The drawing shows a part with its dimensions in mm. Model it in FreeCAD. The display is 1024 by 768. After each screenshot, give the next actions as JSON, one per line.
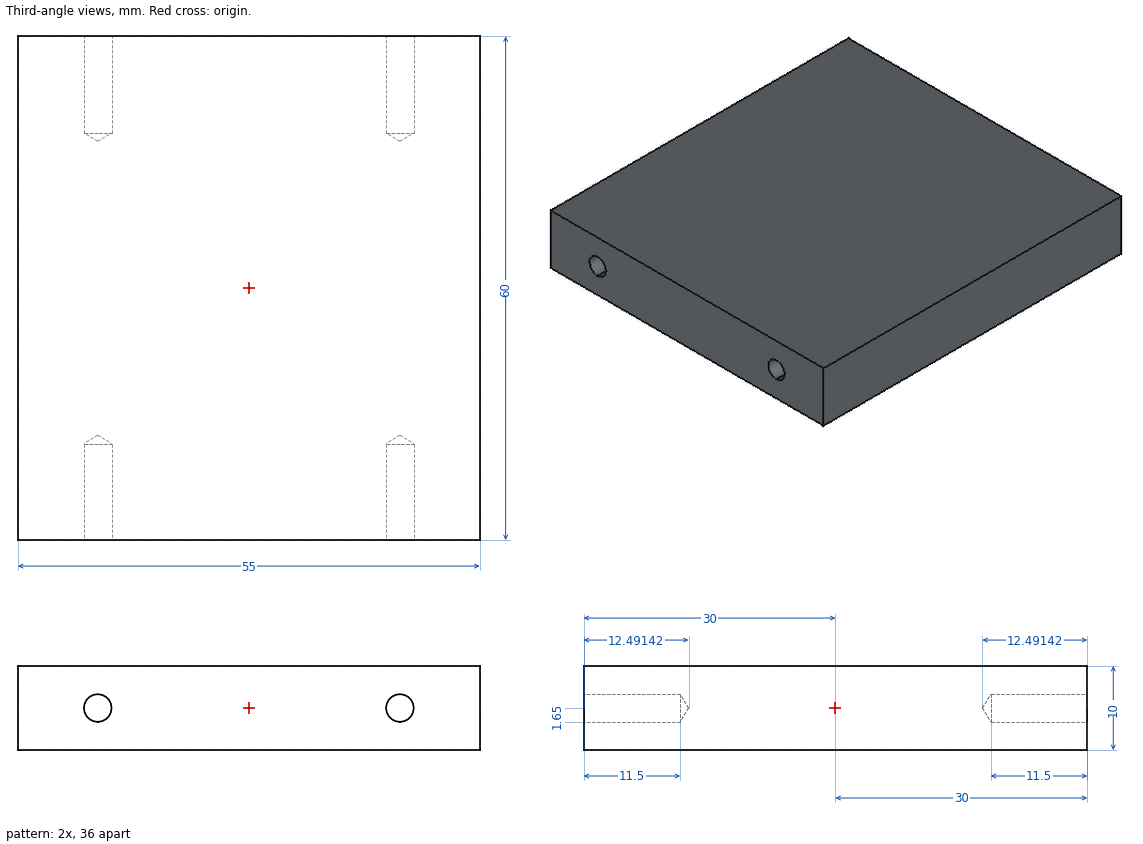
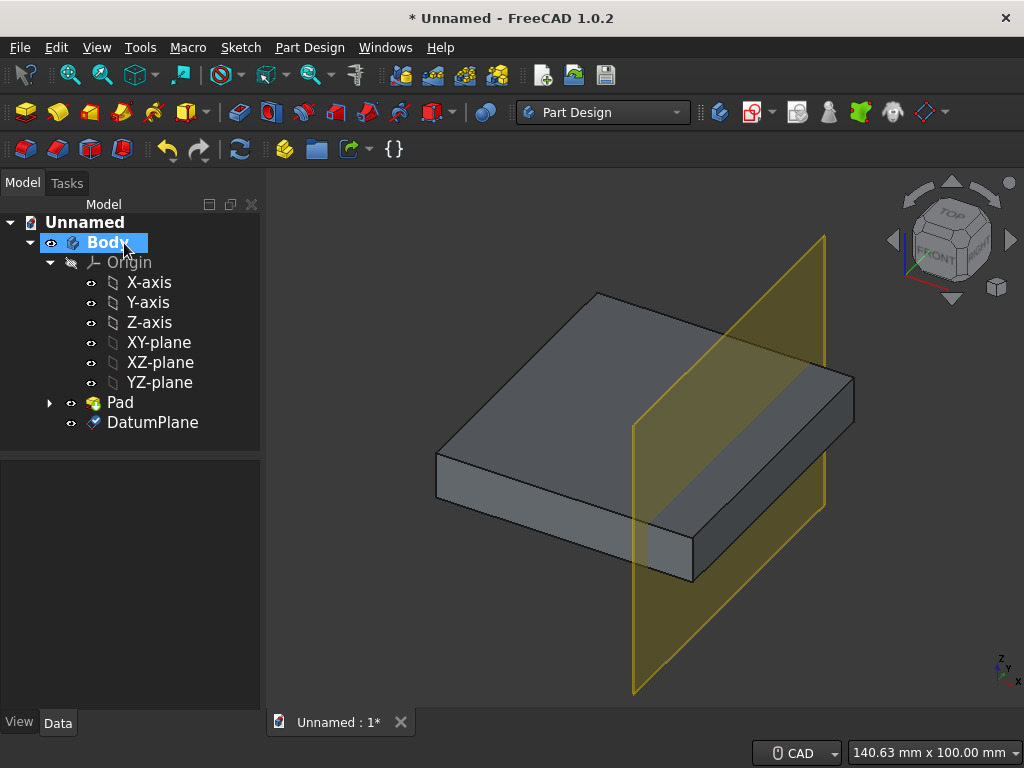
{"action": "left_click", "coordinate": [116, 423]}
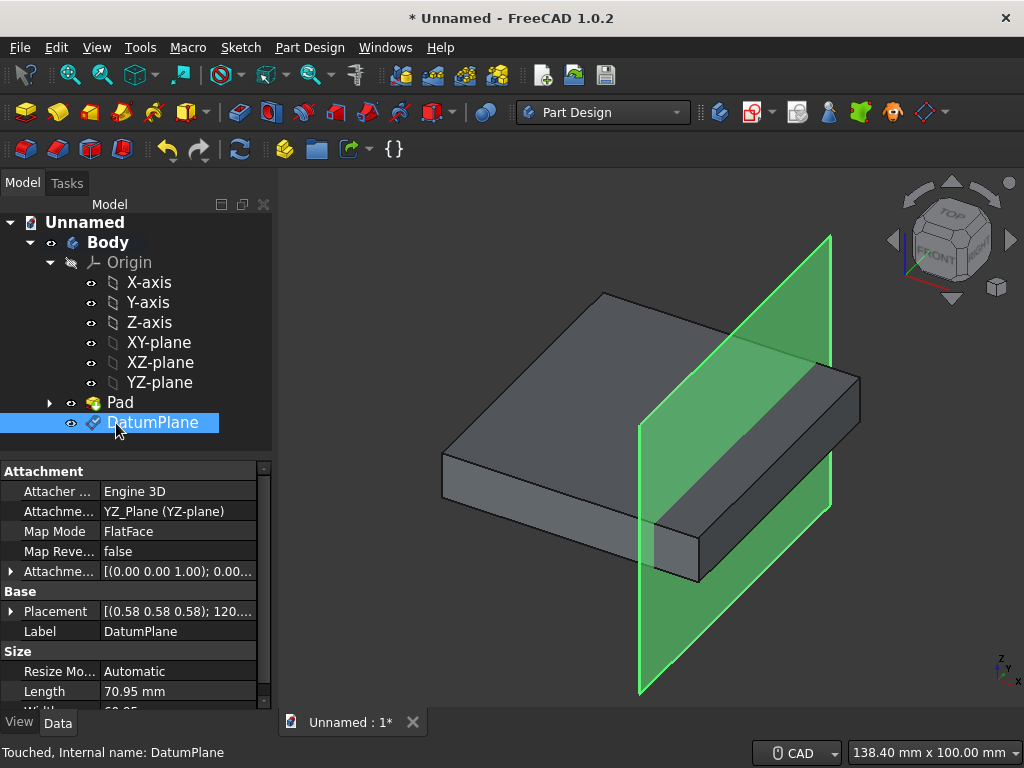
{"action": "left_click", "coordinate": [752, 112]}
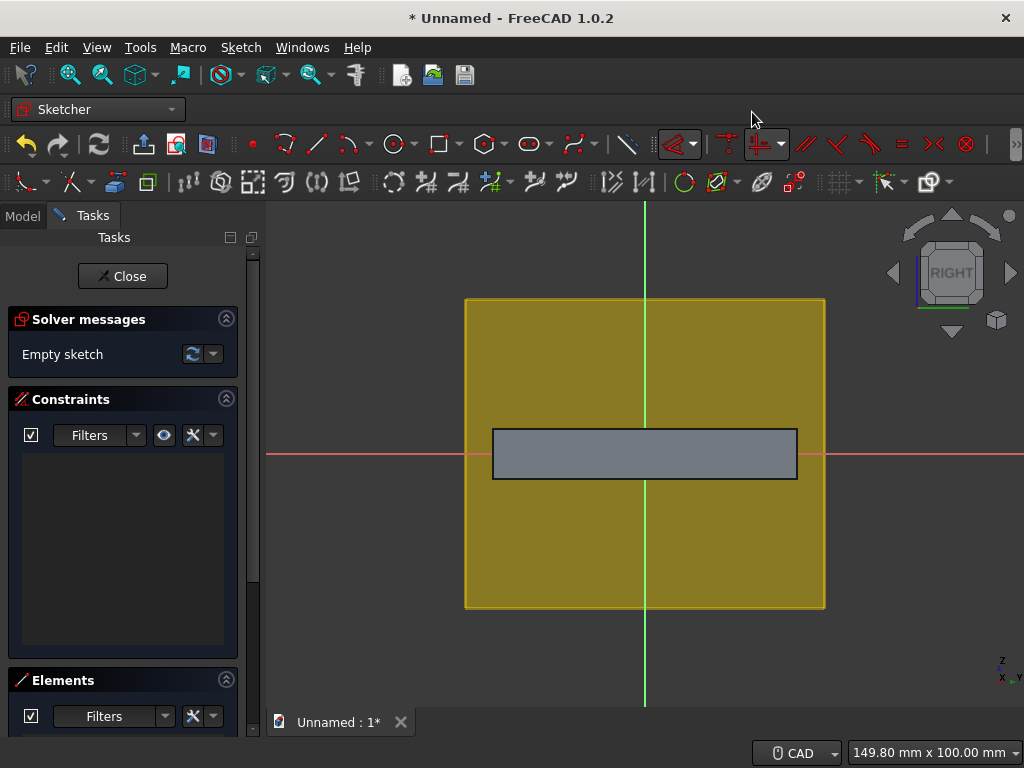
{"action": "left_click", "coordinate": [208, 144]}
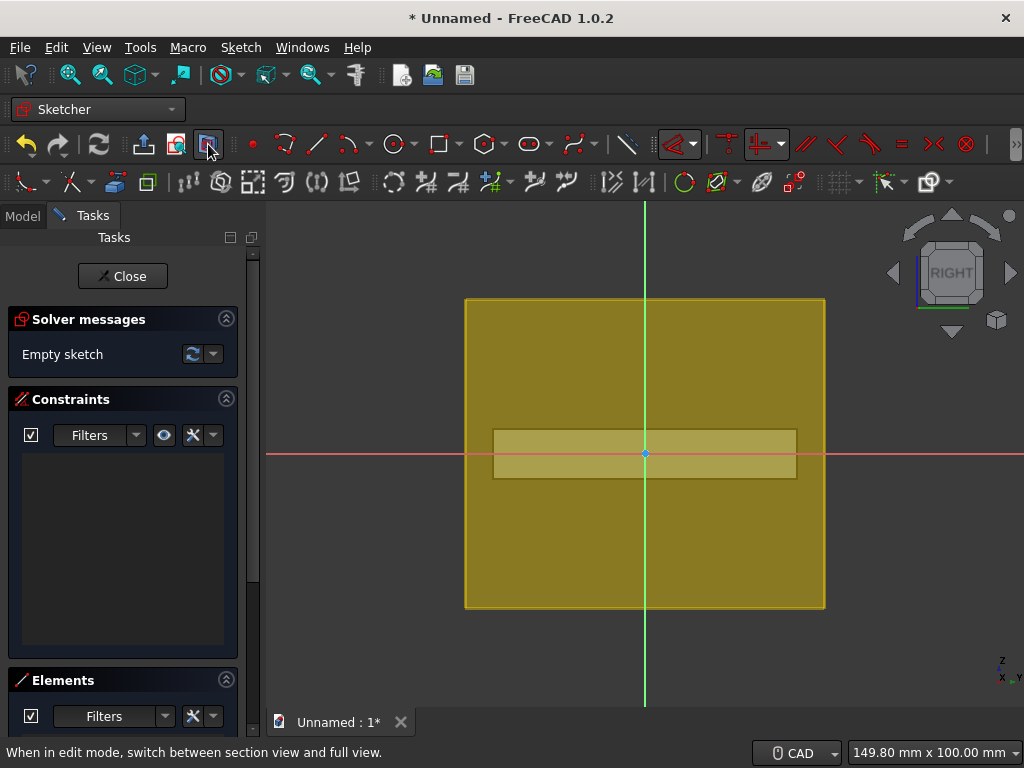
{"action": "scroll", "coordinate": [565, 461], "scroll_direction": "up", "scroll_amount": 5}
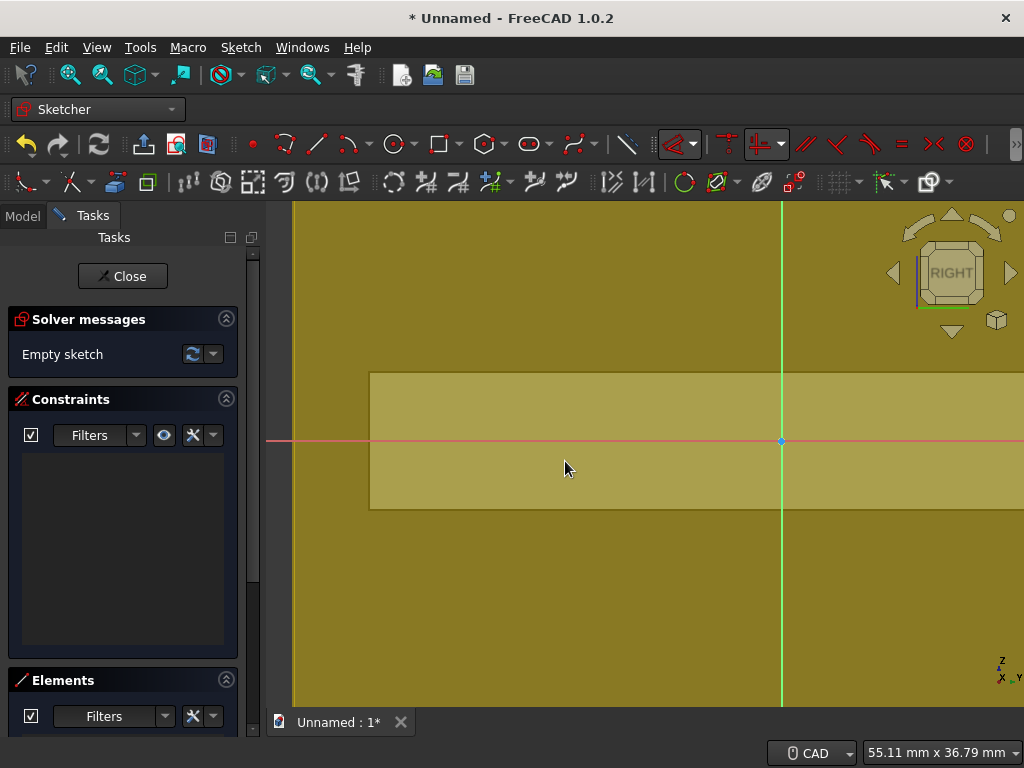
{"action": "key", "text": "g m"}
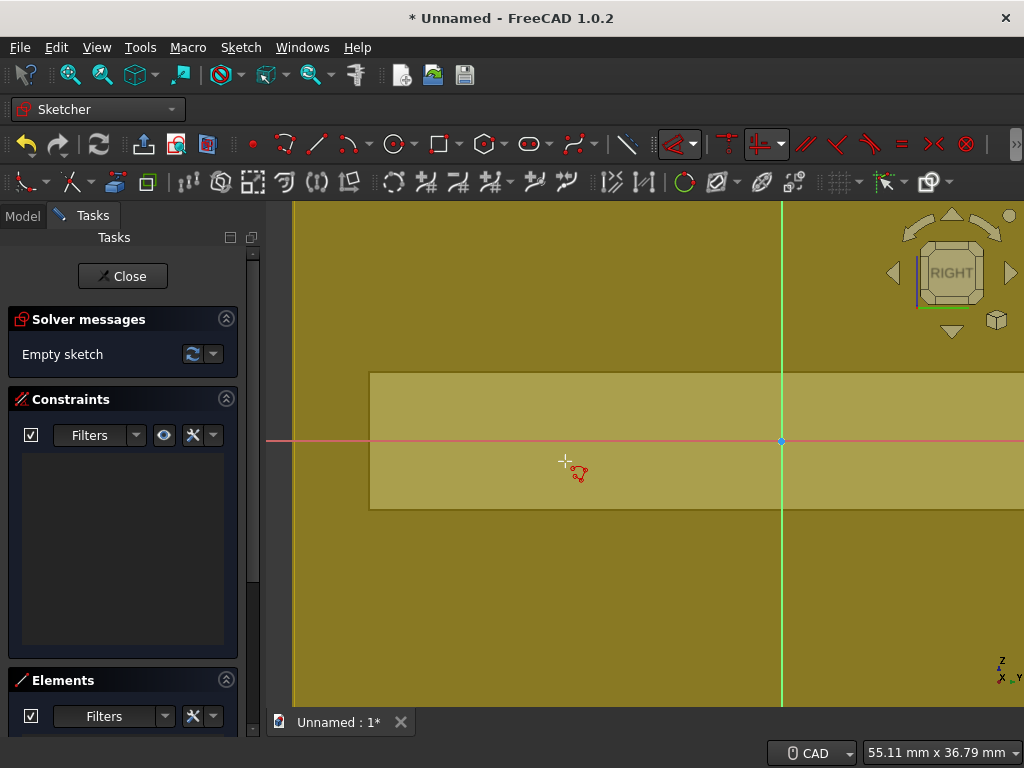
{"action": "left_click", "coordinate": [541, 441]}
{"action": "left_click", "coordinate": [369, 450]}
{"action": "left_click", "coordinate": [369, 464]}
{"action": "left_click", "coordinate": [527, 464]}
{"action": "left_click", "coordinate": [541, 441]}
{"action": "key", "text": "Escape"}
{"action": "key", "text": "Escape"}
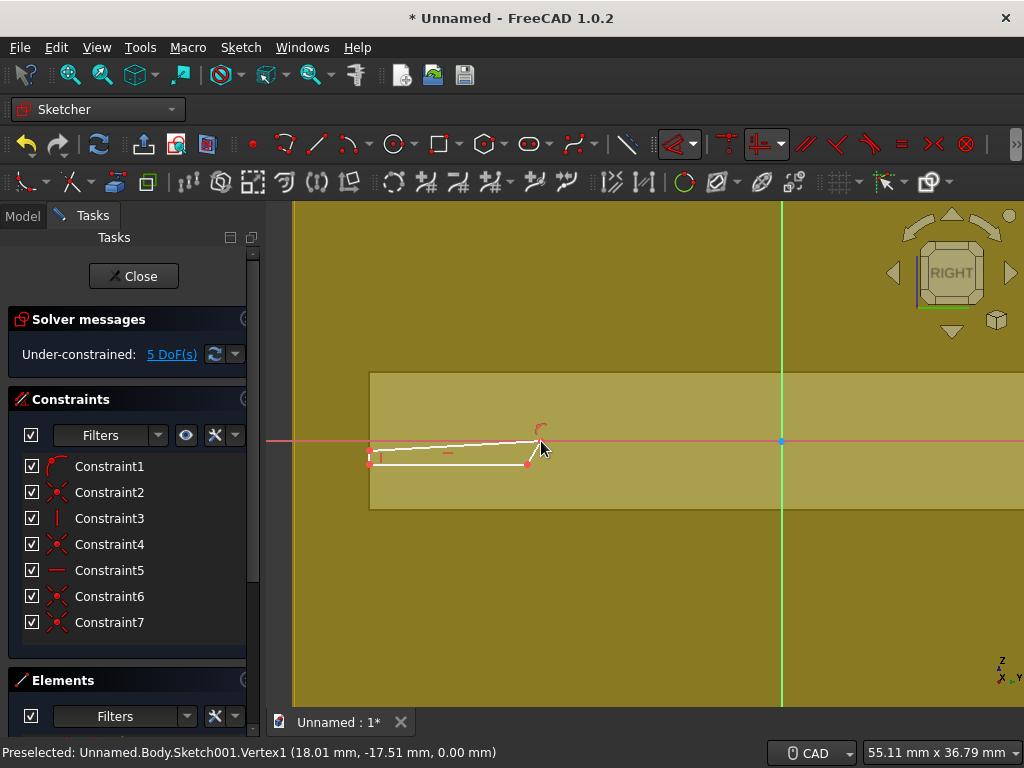
{"action": "left_click", "coordinate": [489, 444]}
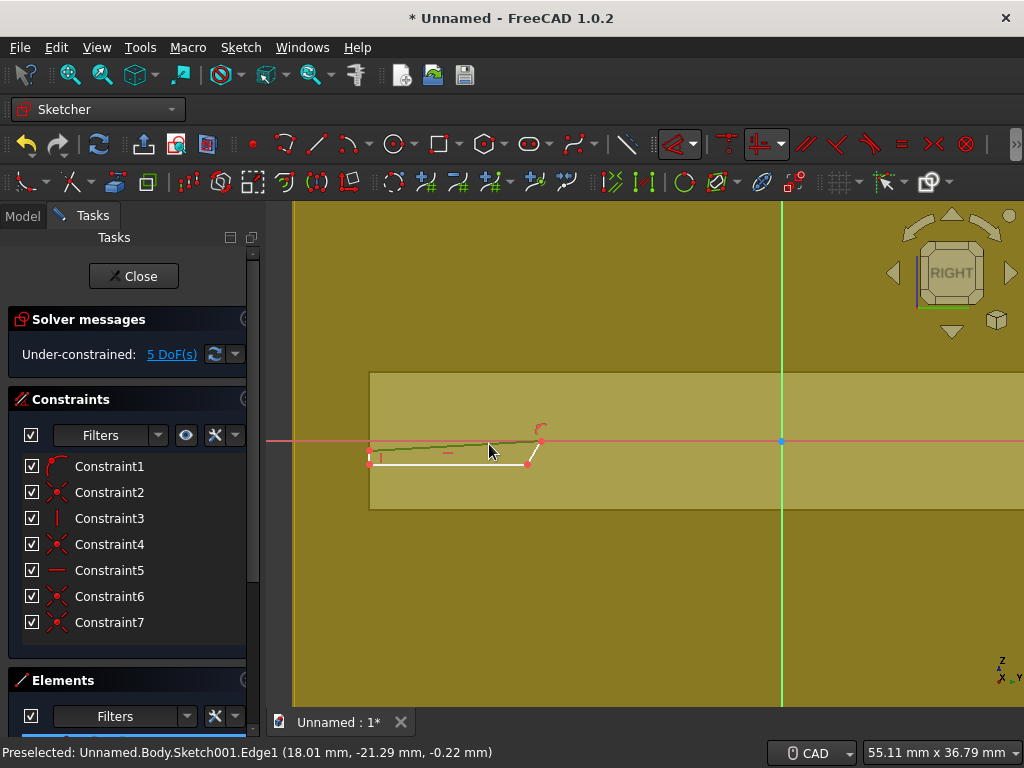
{"action": "key", "text": "h"}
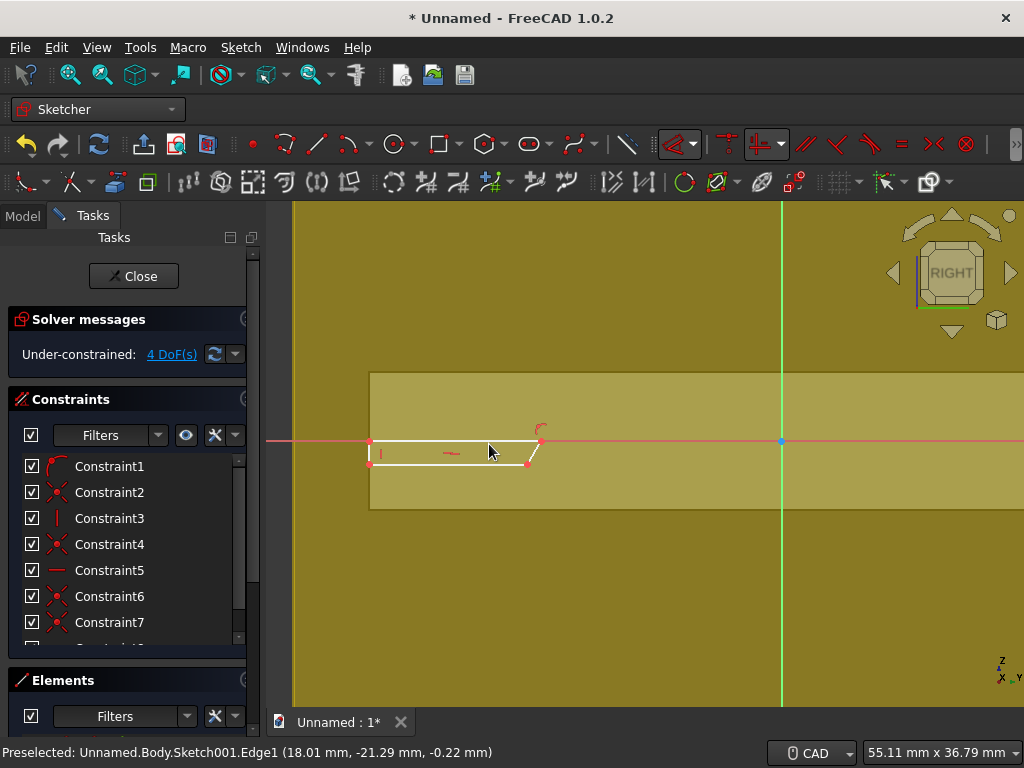
{"action": "left_click", "coordinate": [674, 144]}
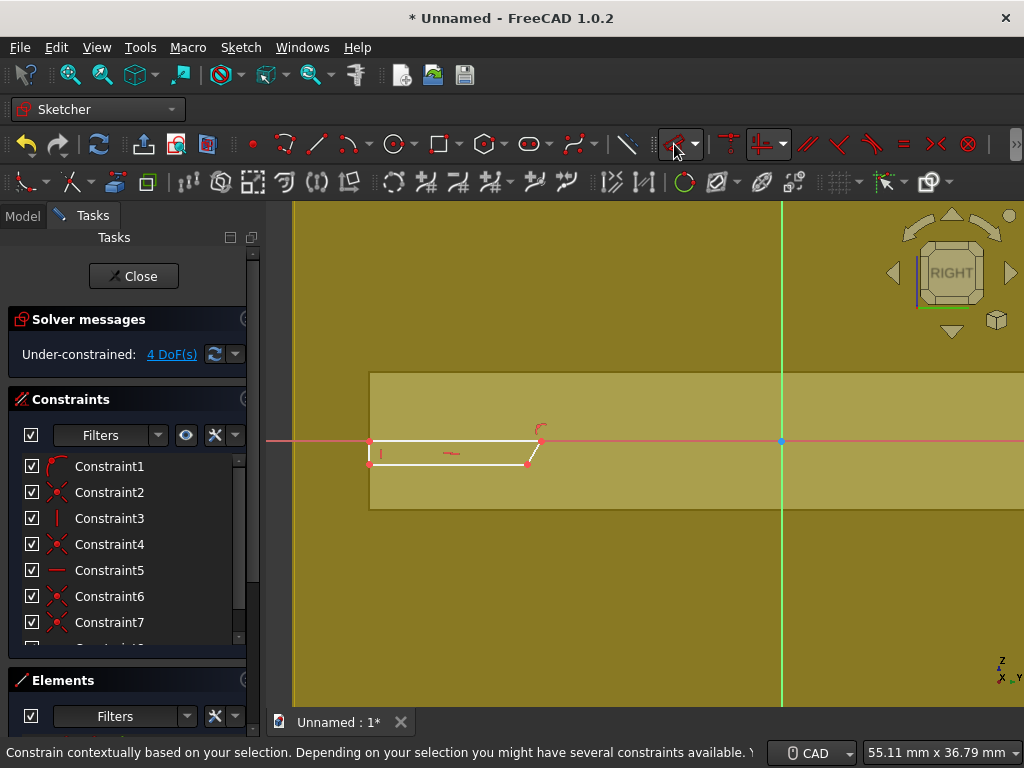
{"action": "left_click", "coordinate": [369, 441]}
{"action": "left_click", "coordinate": [575, 407]}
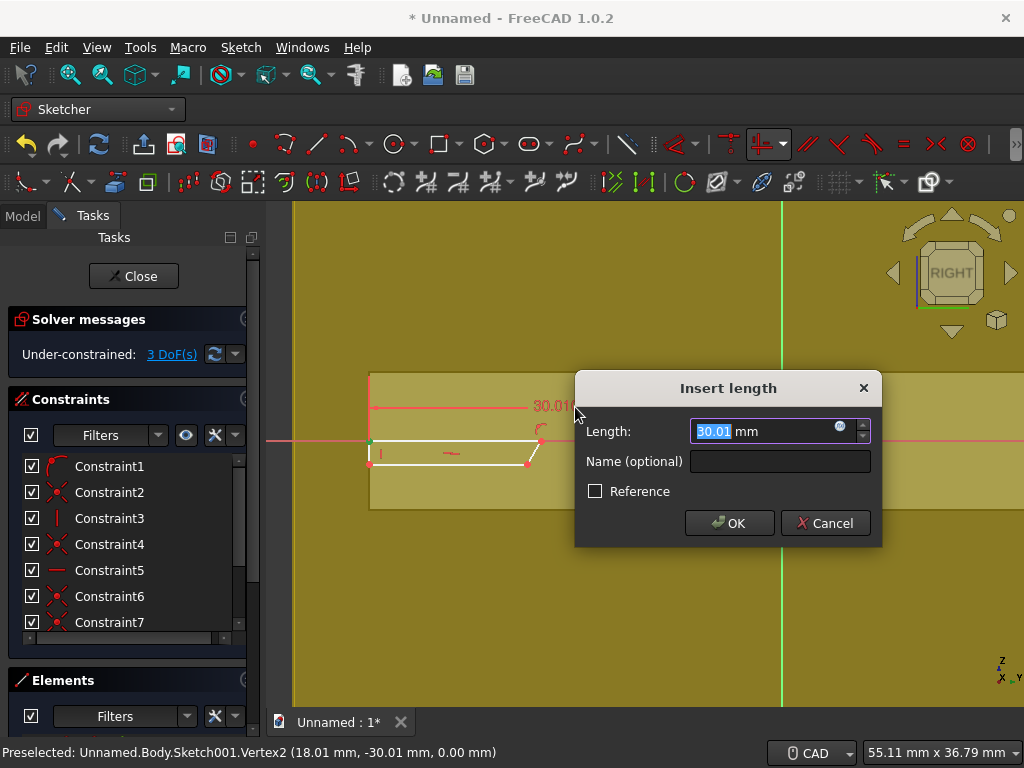
{"action": "type", "text": "30"}
{"action": "key", "text": "Return"}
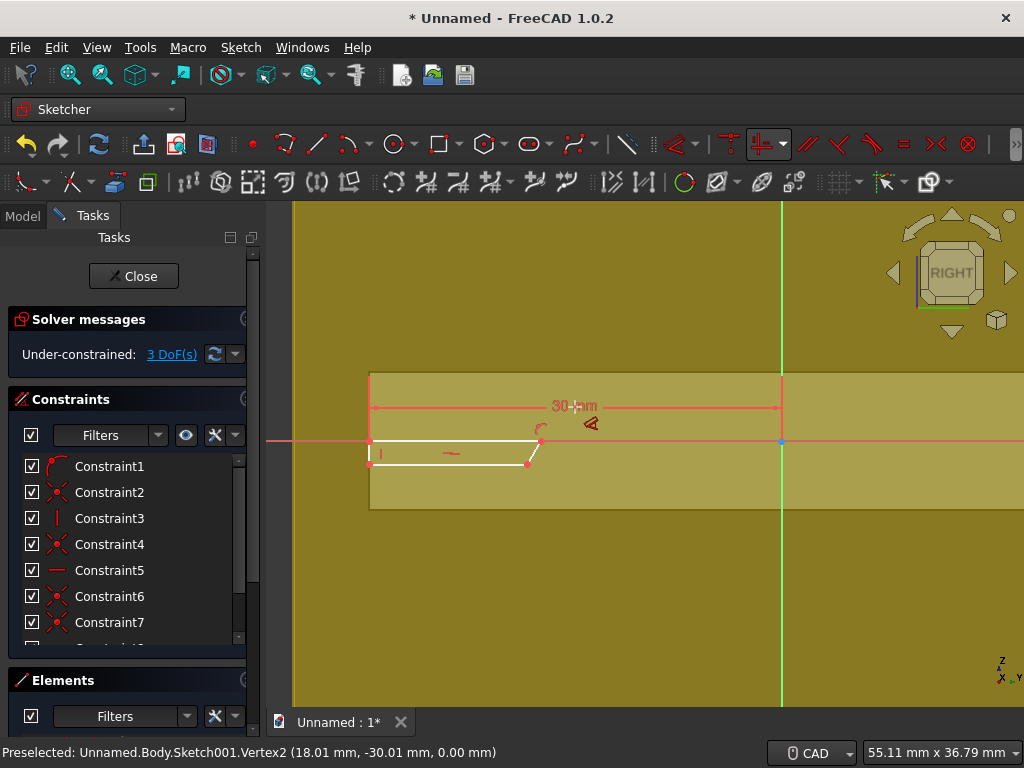
{"action": "scroll", "coordinate": [369, 451], "scroll_direction": "up", "scroll_amount": 3}